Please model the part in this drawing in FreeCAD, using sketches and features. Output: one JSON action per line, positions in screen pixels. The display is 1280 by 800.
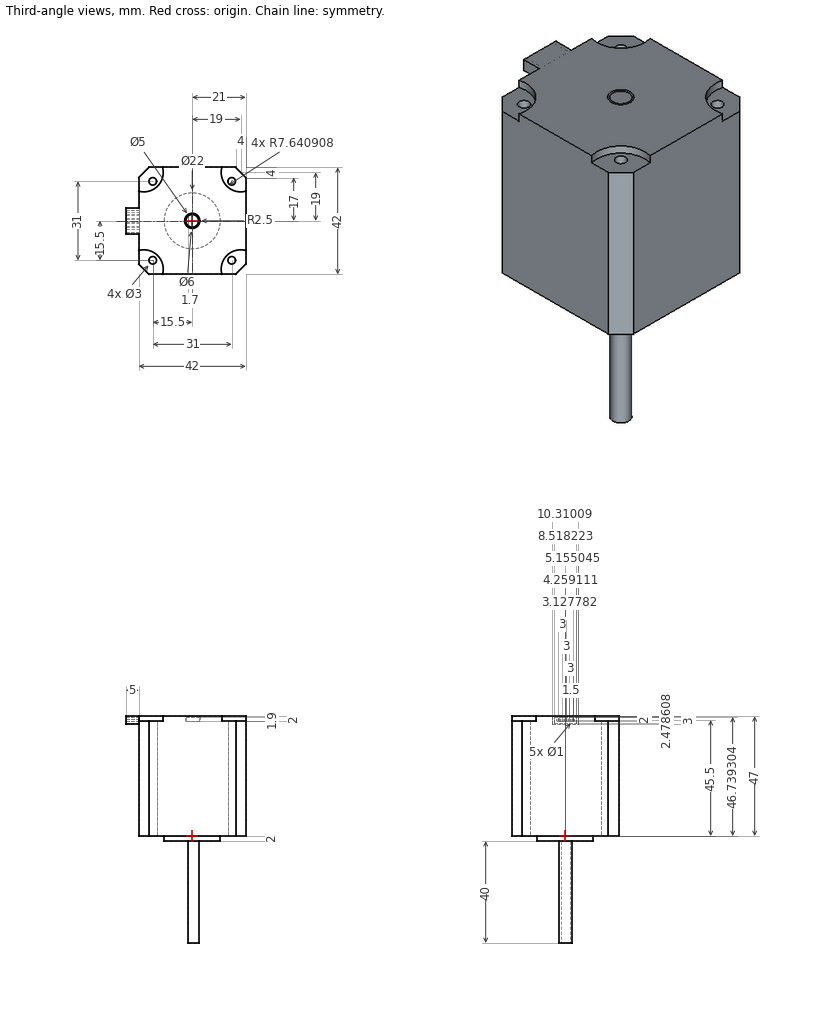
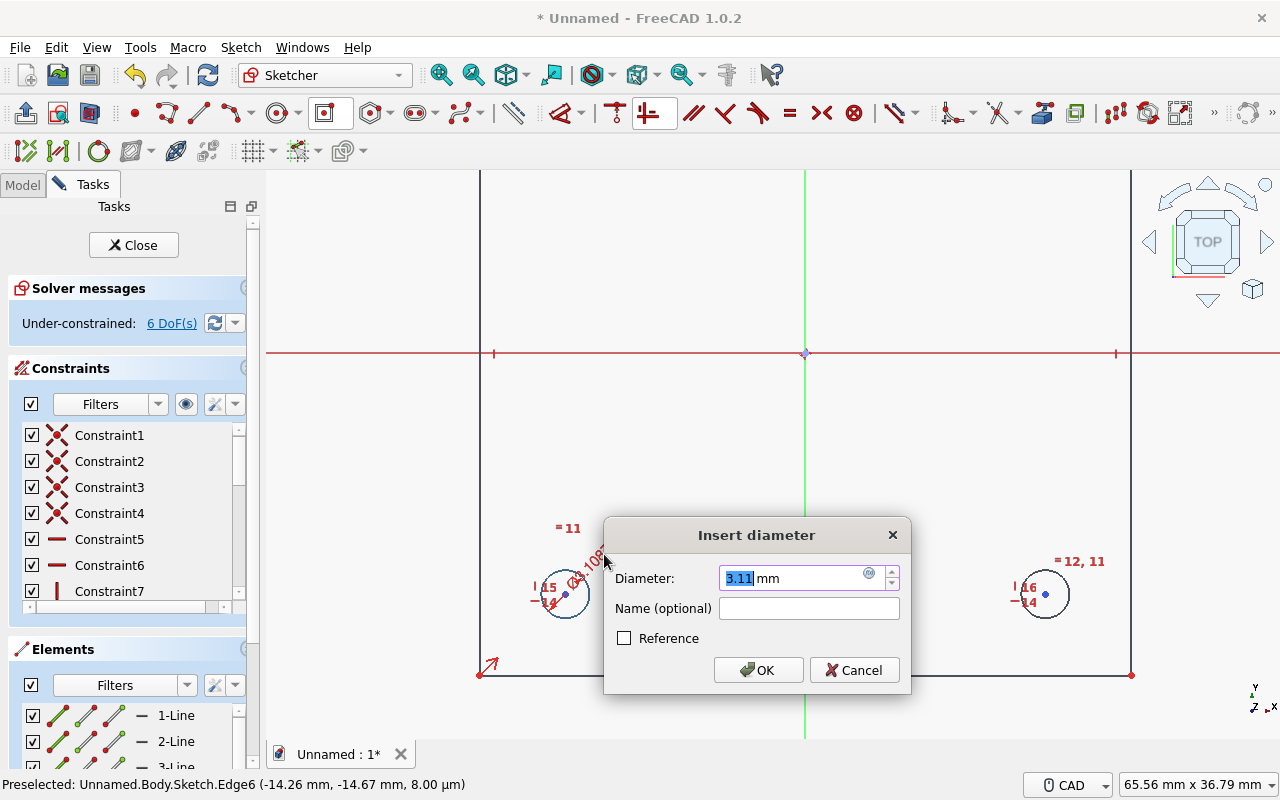
{"action": "type", "text": "3"}
{"action": "key", "text": "Return"}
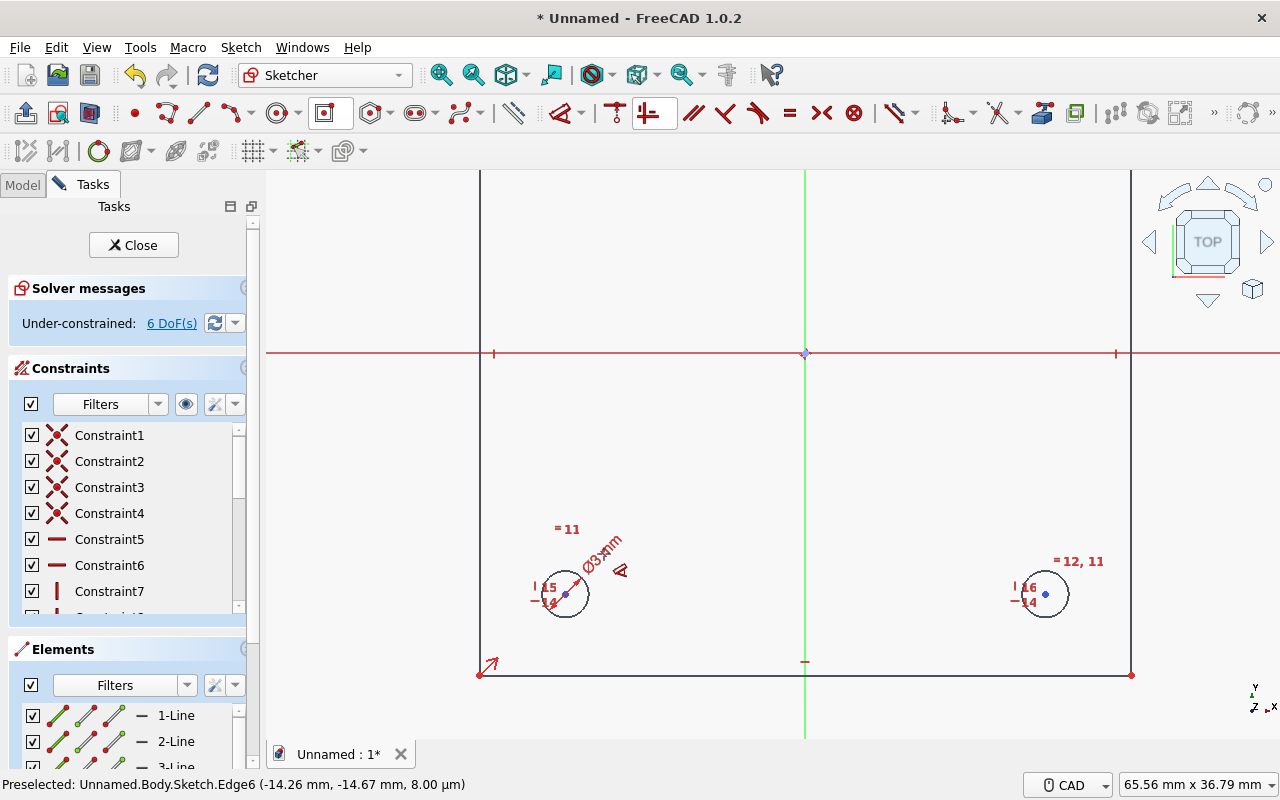
{"action": "left_click", "coordinate": [675, 676]}
{"action": "left_click", "coordinate": [651, 710]}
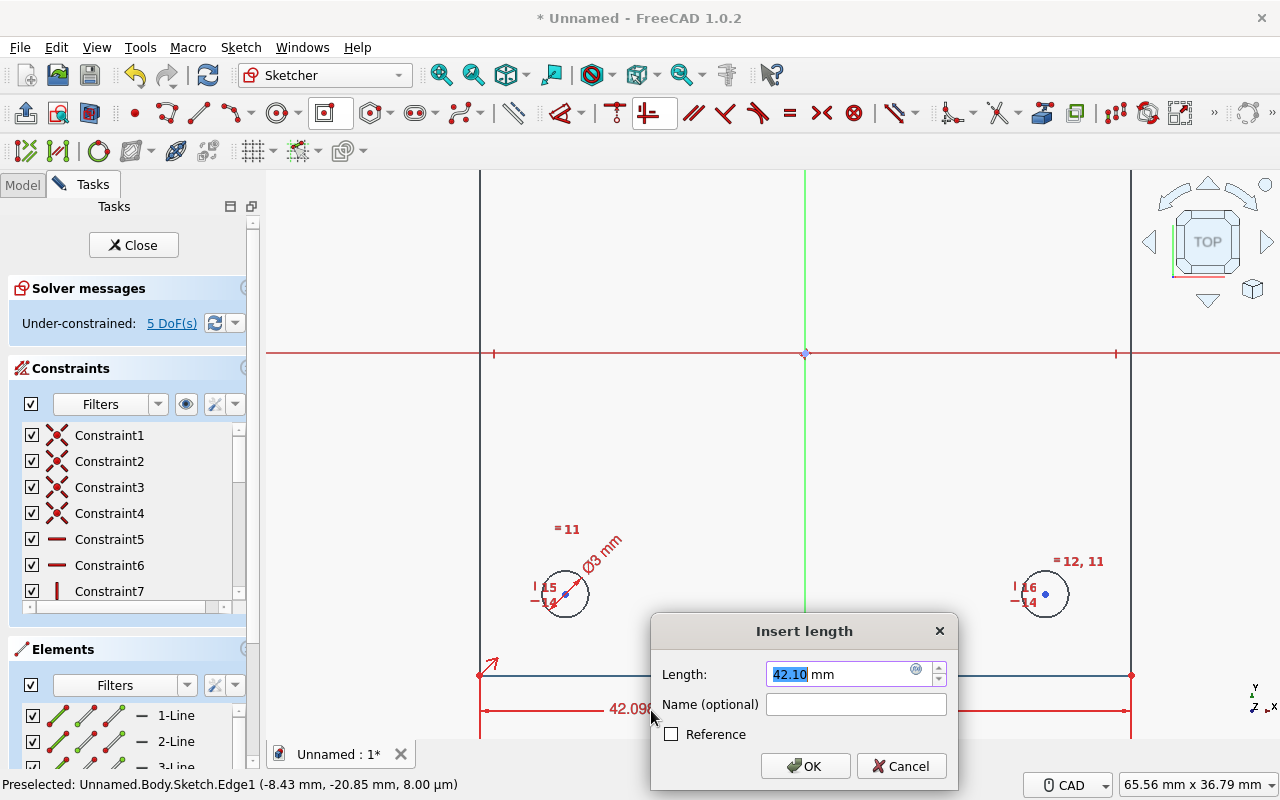
{"action": "type", "text": "42"}
{"action": "key", "text": "Return"}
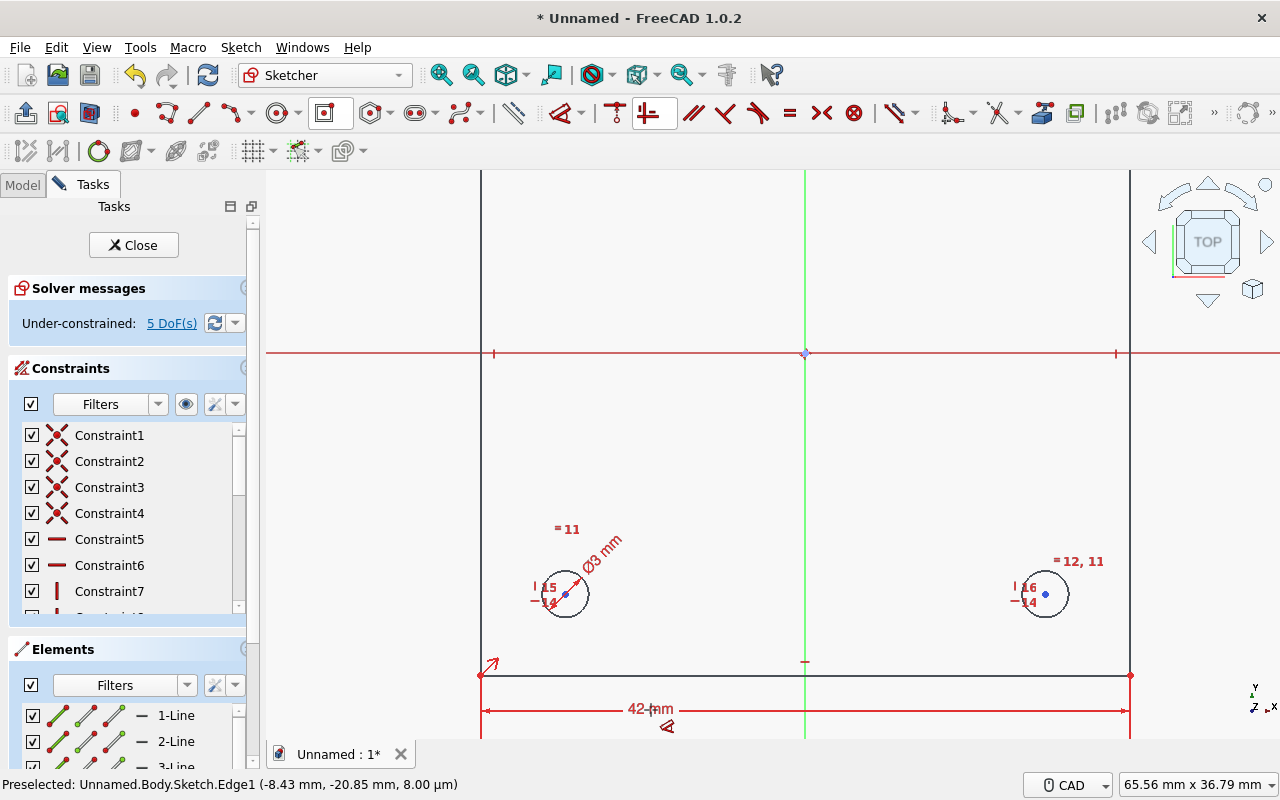
{"action": "scroll", "coordinate": [582, 578], "scroll_direction": "down", "scroll_amount": 3}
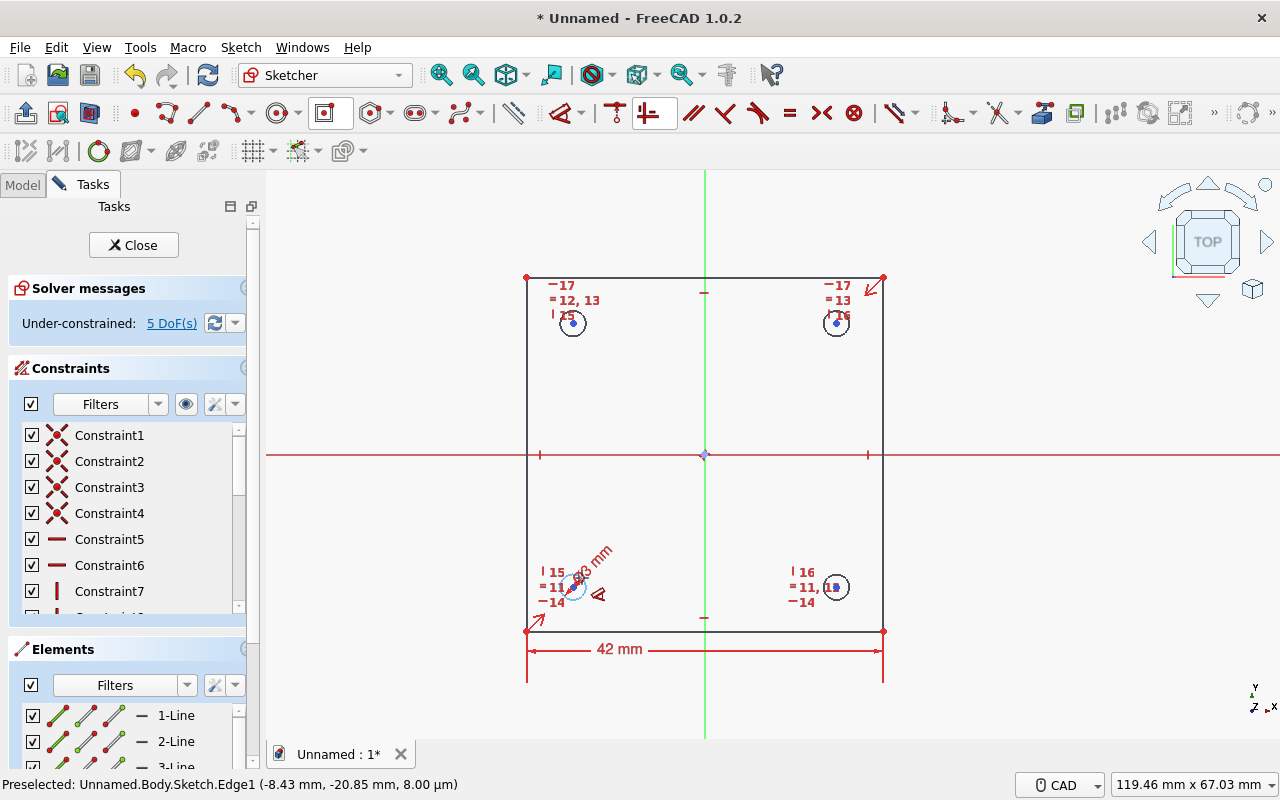
{"action": "left_click", "coordinate": [883, 526]}
{"action": "left_click", "coordinate": [917, 373]}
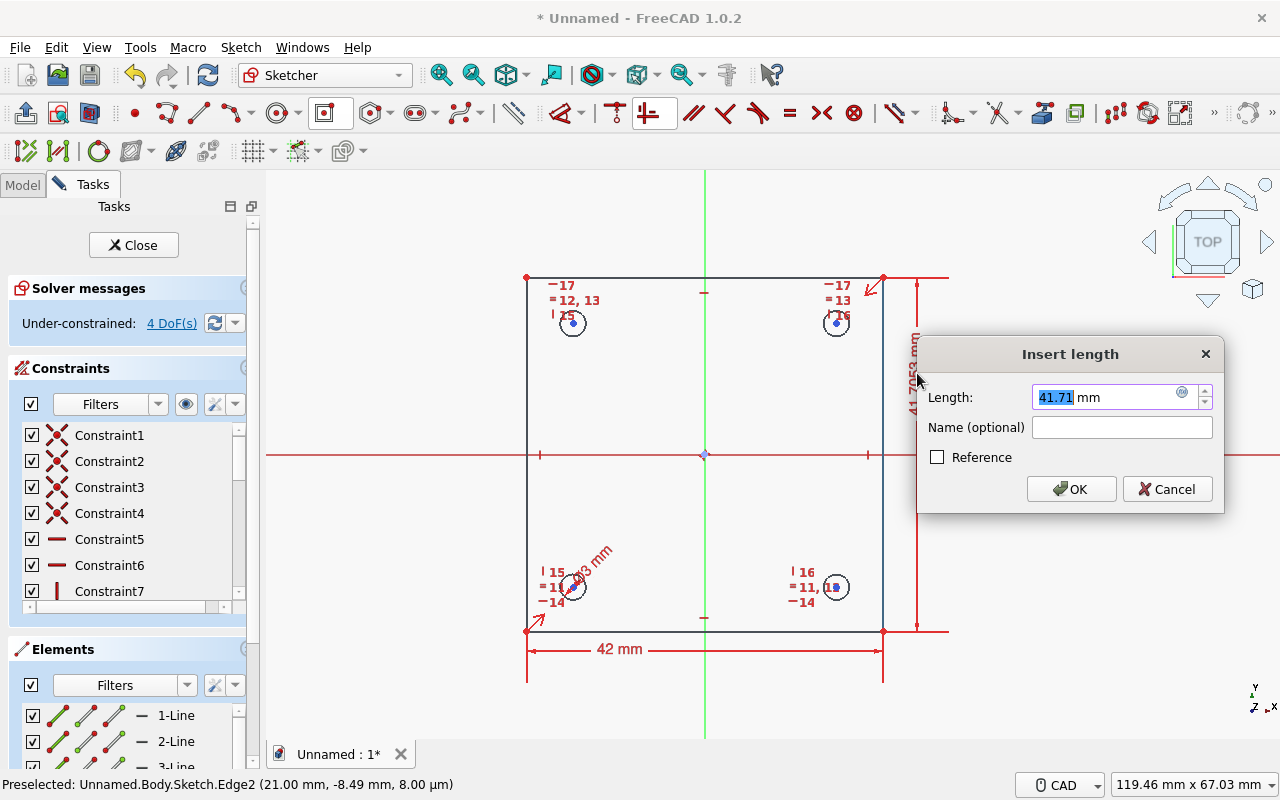
{"action": "type", "text": "42"}
{"action": "key", "text": "Return"}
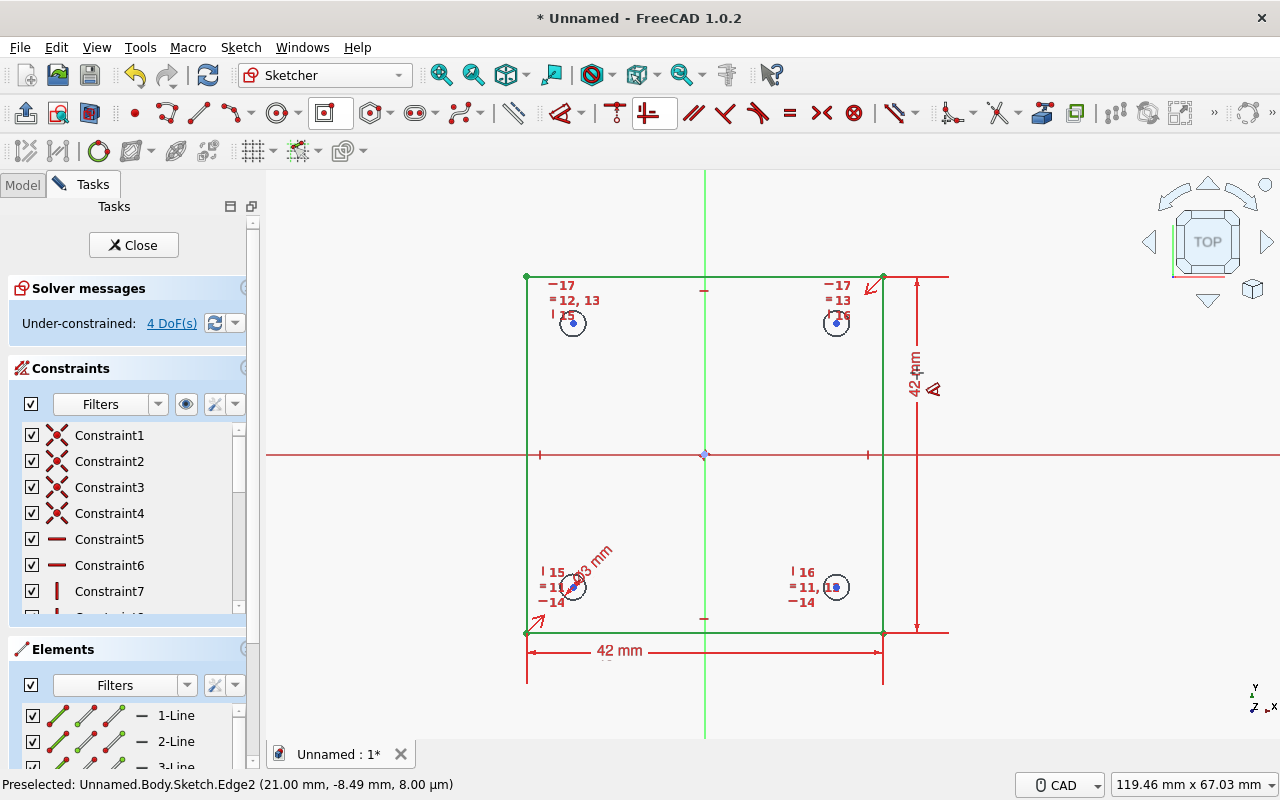
{"action": "left_click", "coordinate": [573, 587]}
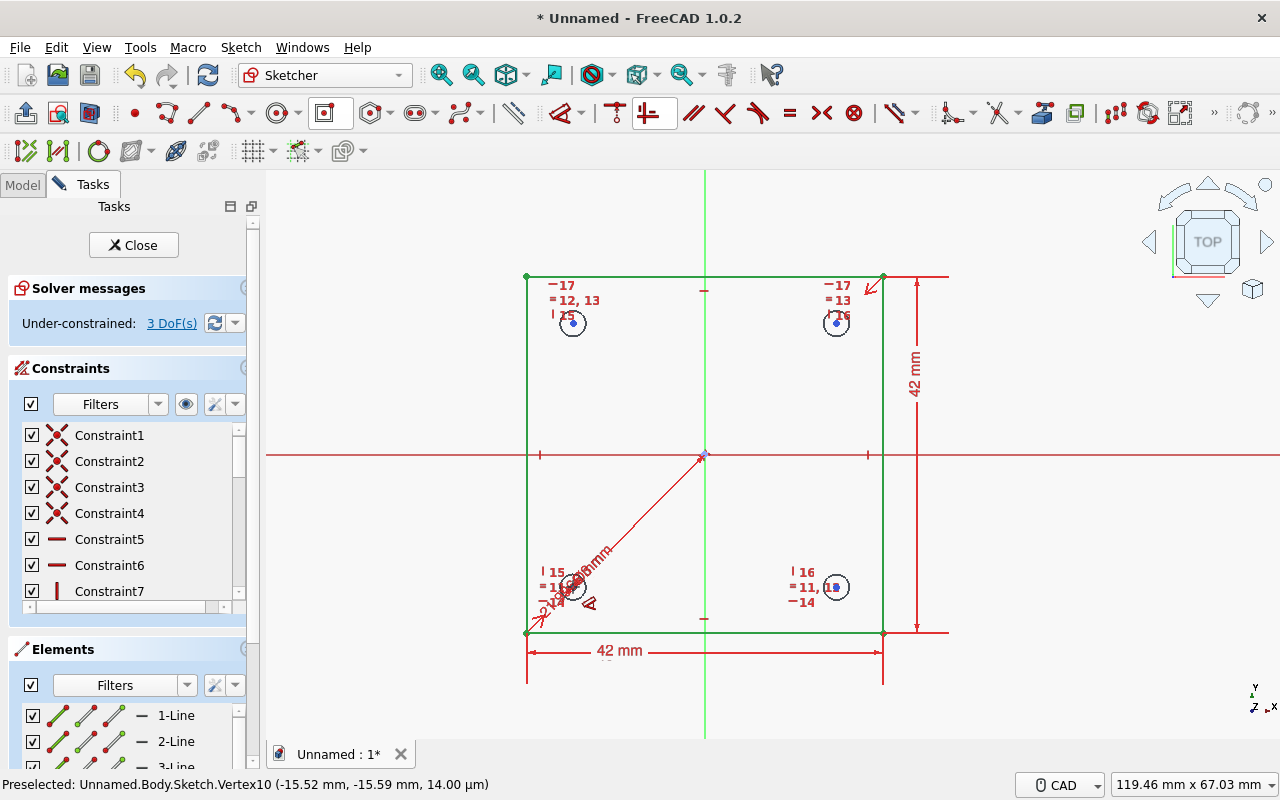
{"action": "left_click", "coordinate": [836, 587]}
{"action": "left_click", "coordinate": [765, 553]}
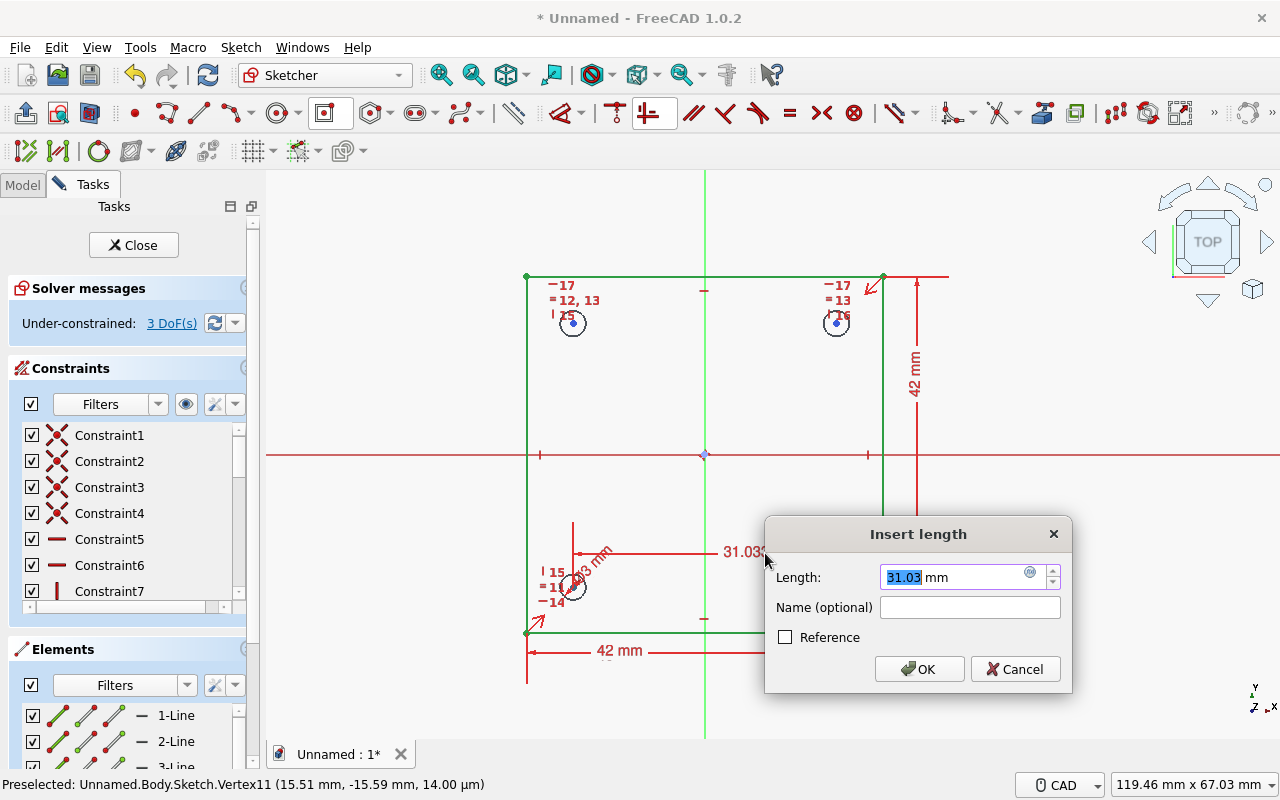
{"action": "type", "text": "31"}
{"action": "key", "text": "Return"}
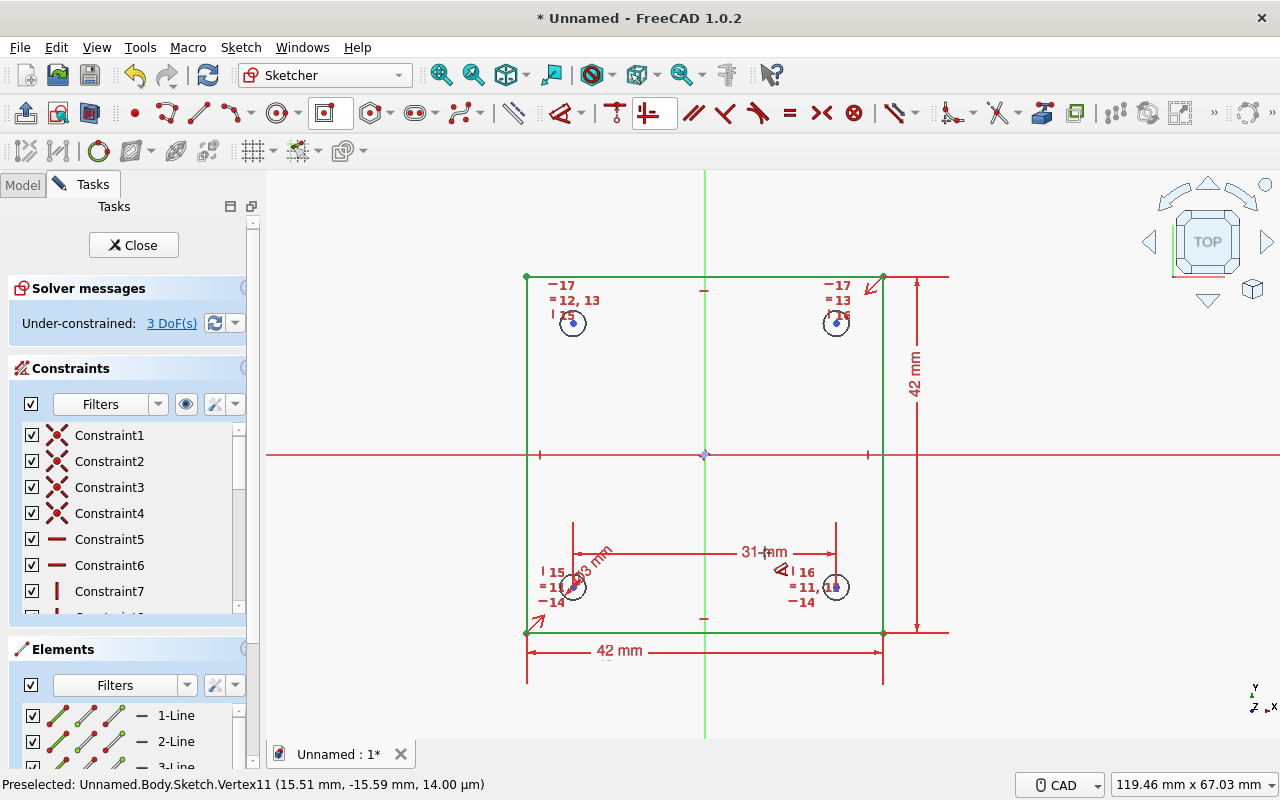
{"action": "left_click", "coordinate": [573, 587]}